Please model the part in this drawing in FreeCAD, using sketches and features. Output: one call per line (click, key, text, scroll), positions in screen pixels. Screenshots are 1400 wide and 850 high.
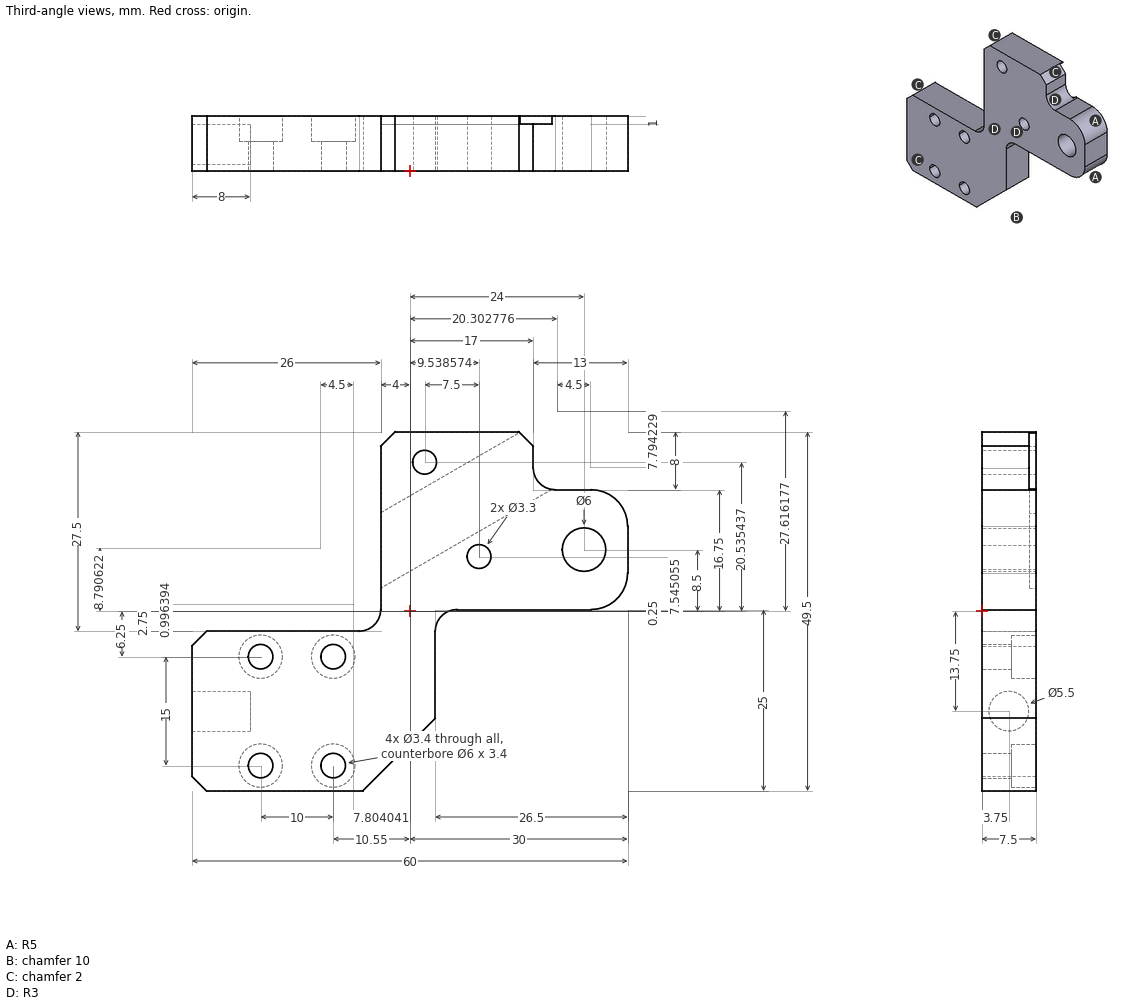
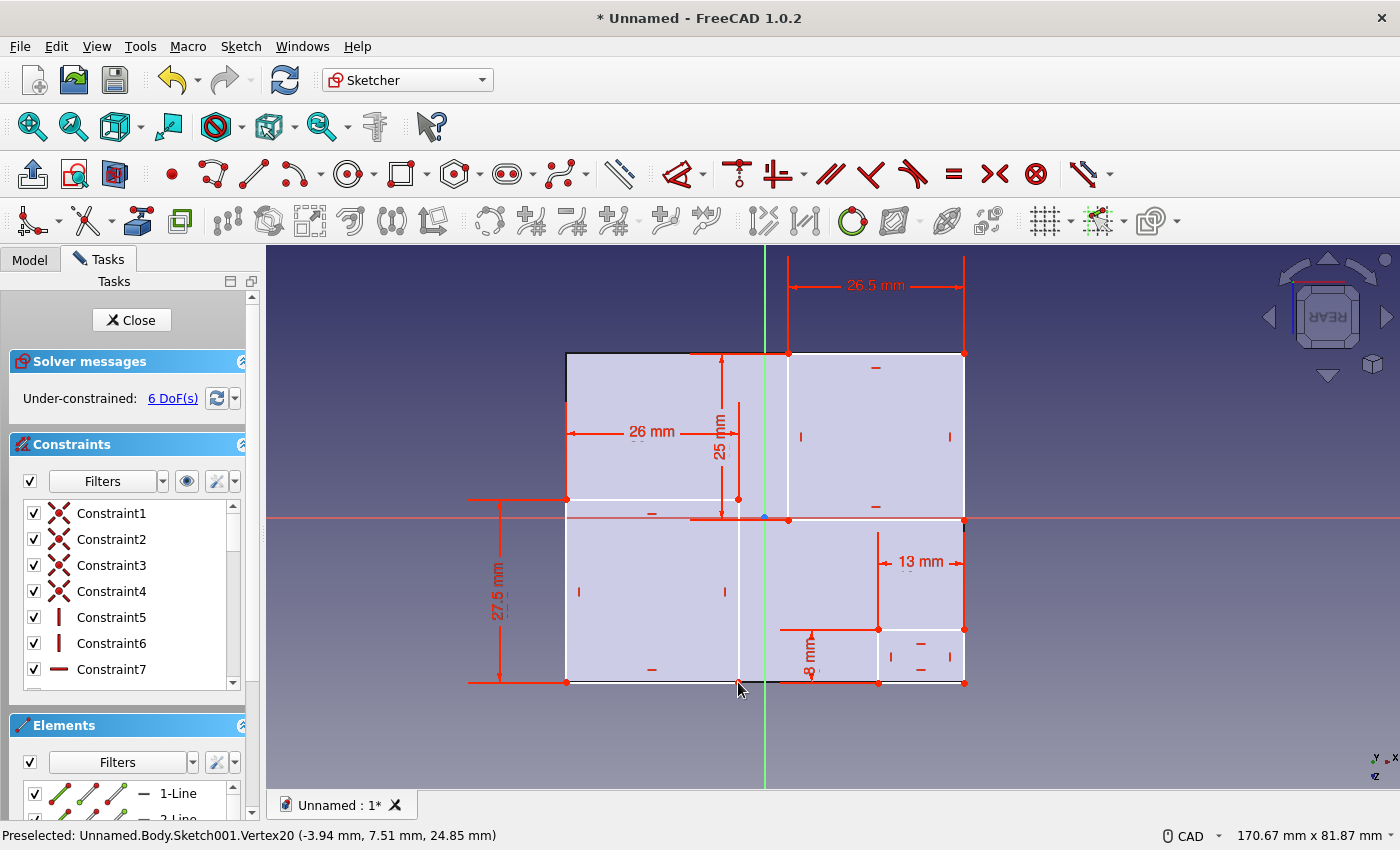
click(676, 174)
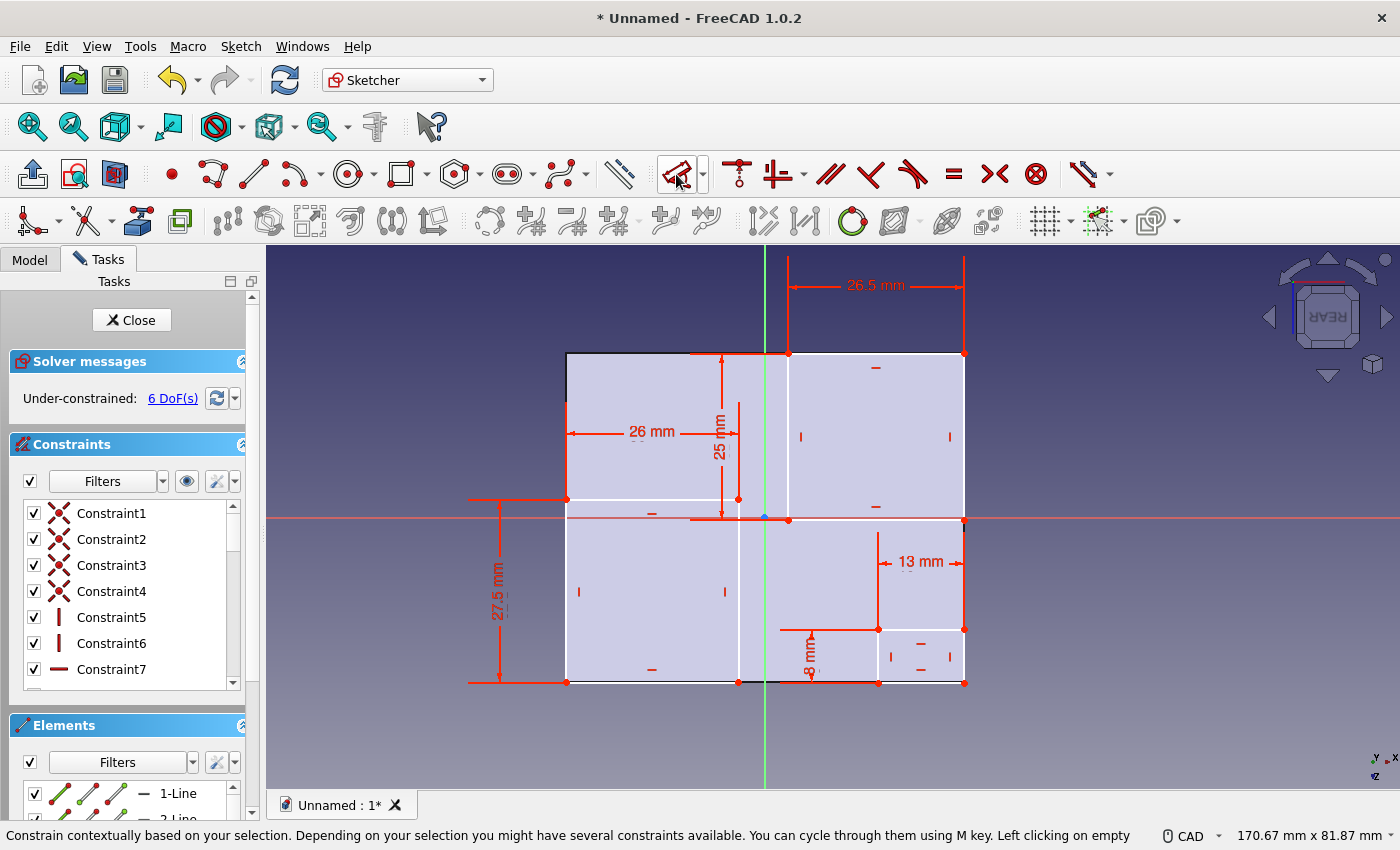
scroll(739, 683, up, 3)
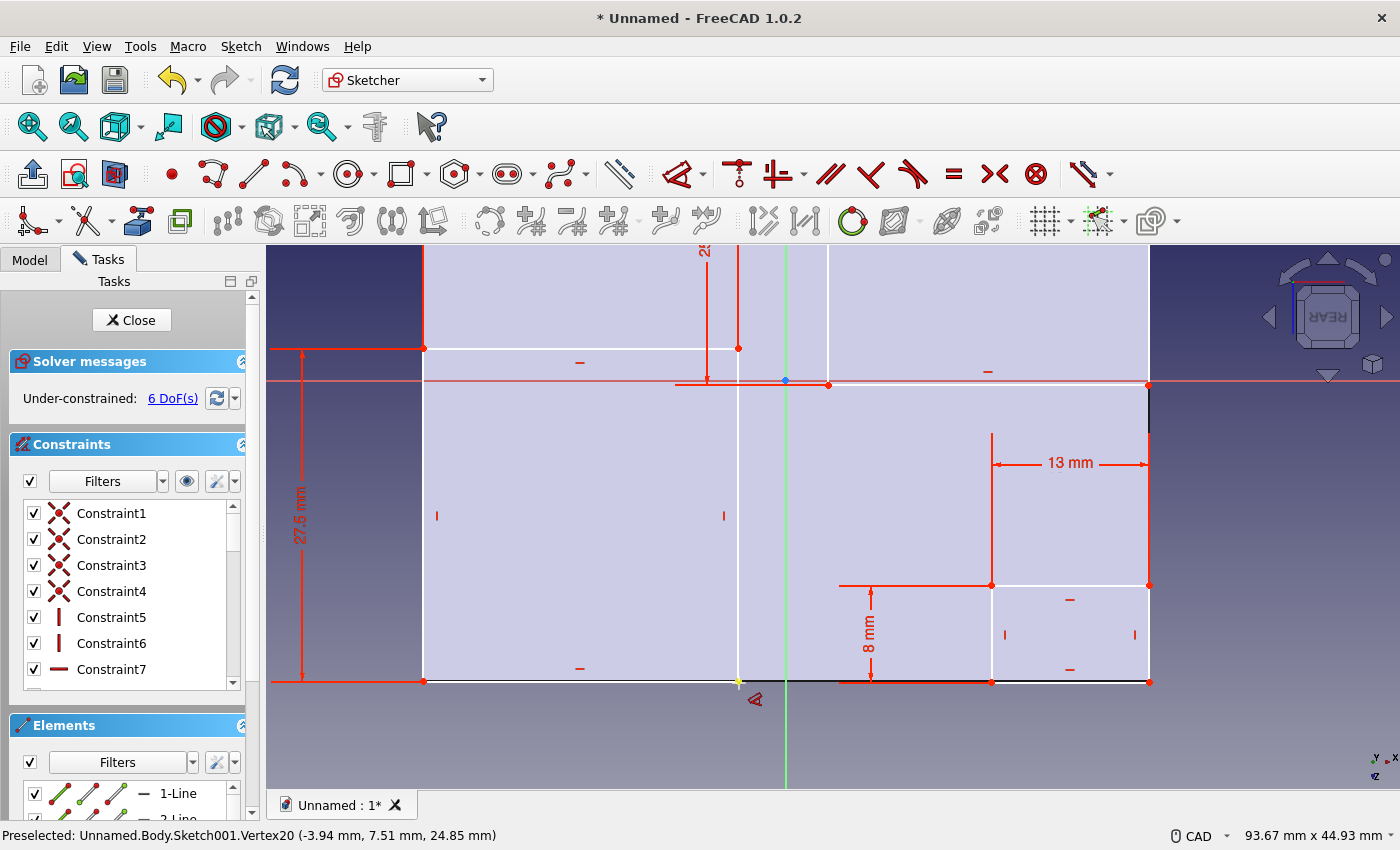
click(738, 682)
click(762, 716)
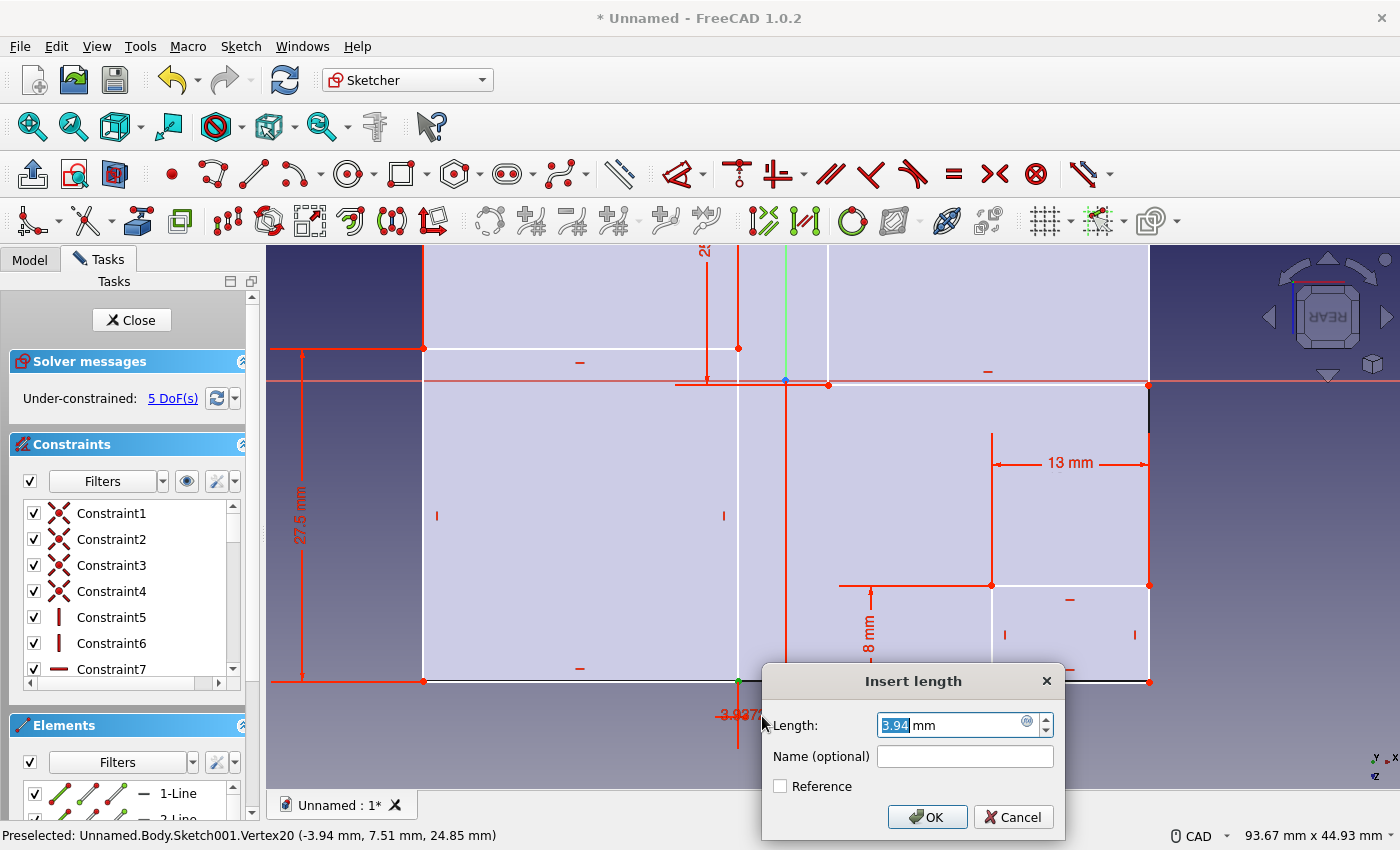
text(4)
key(Return)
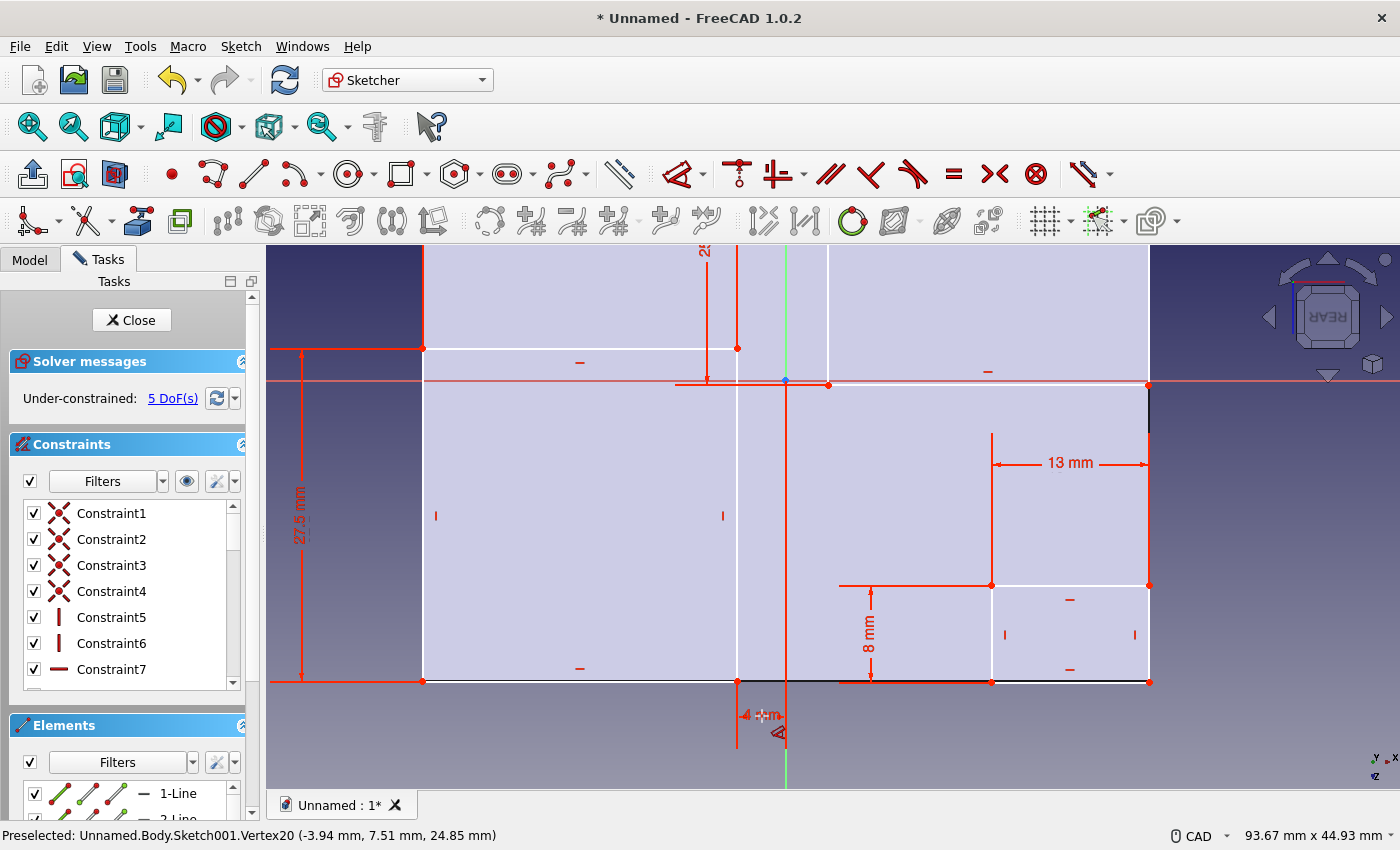
click(1149, 385)
click(967, 419)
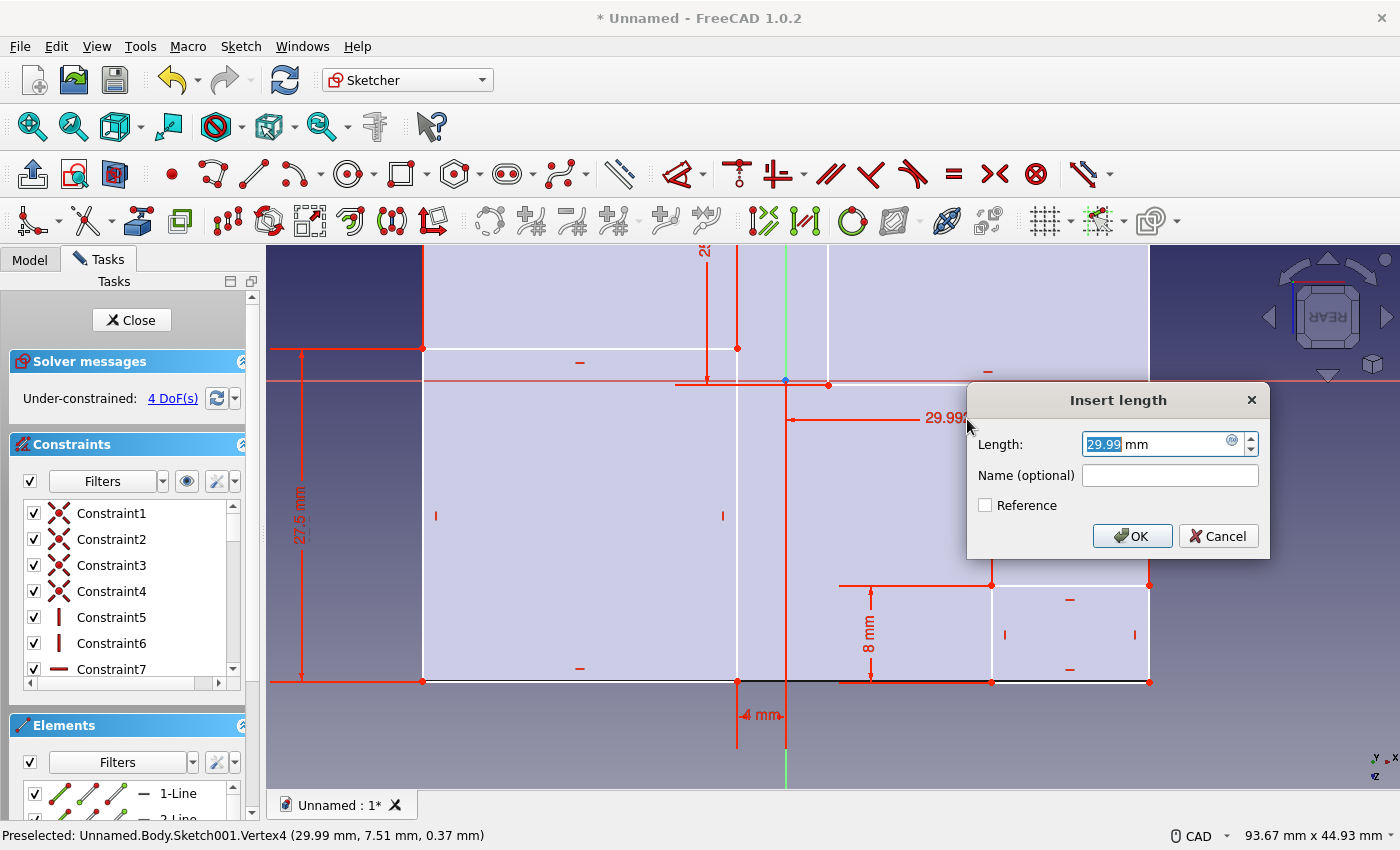
text(30)
key(Return)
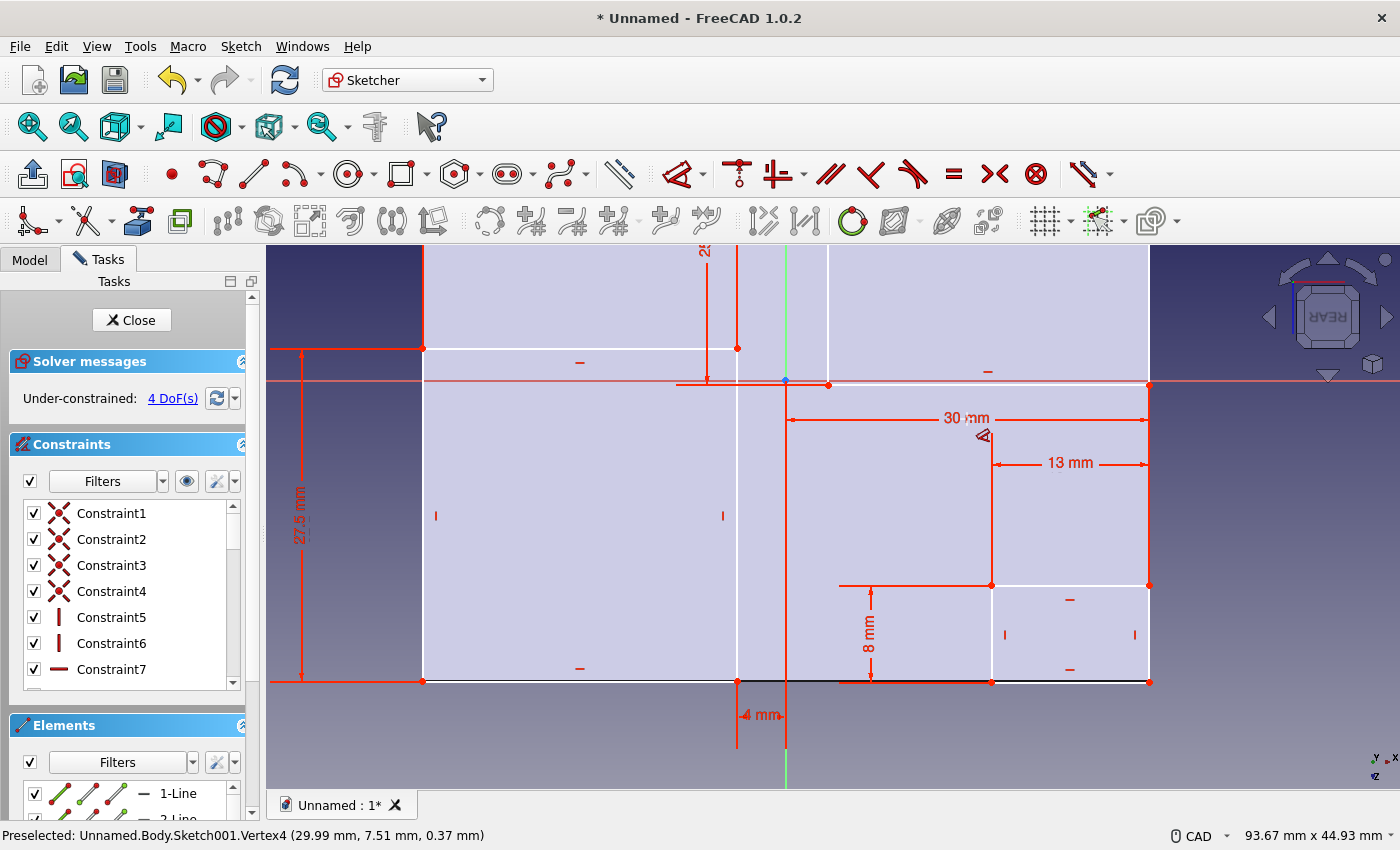
click(992, 586)
click(889, 620)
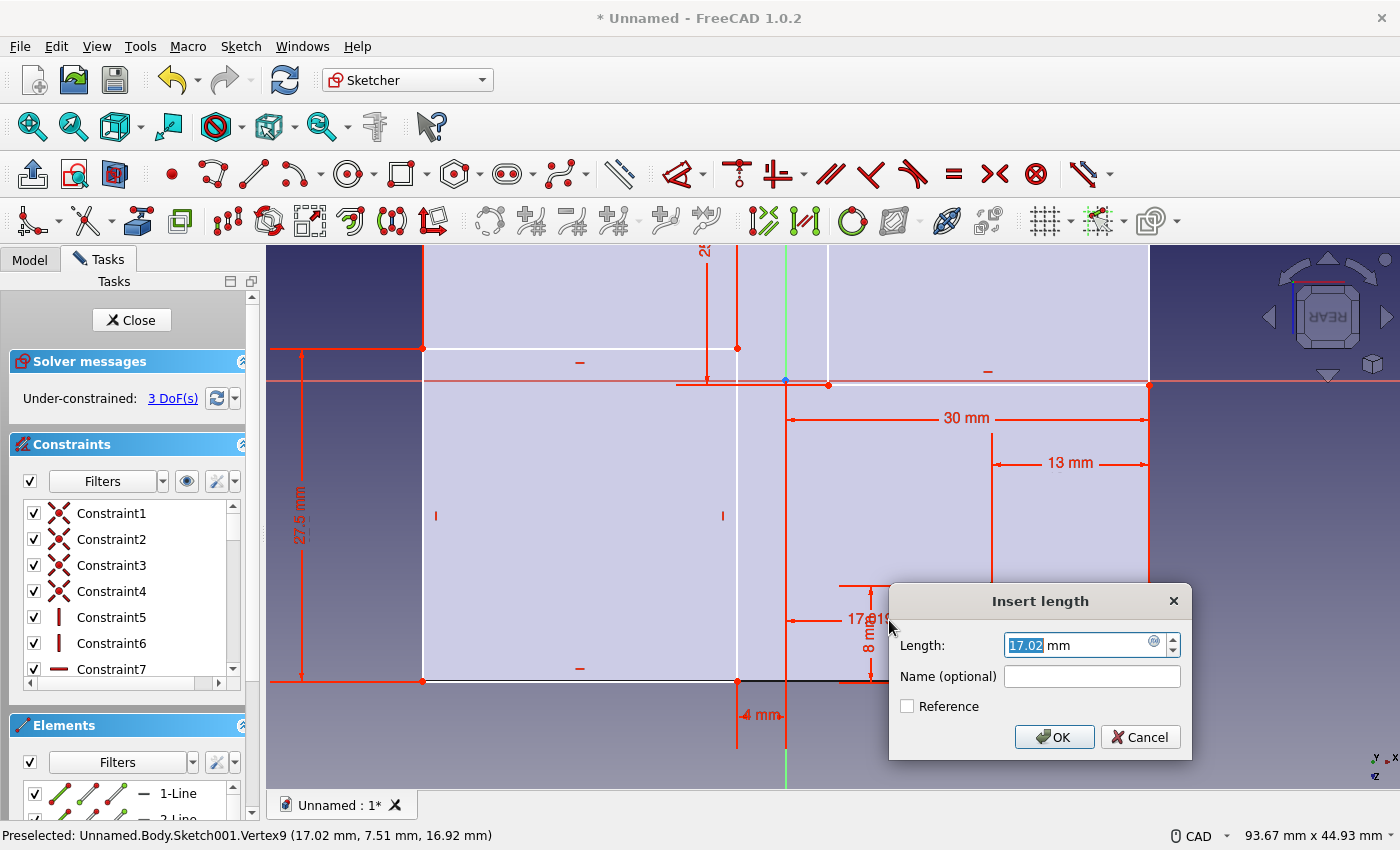
text(17)
key(Return)